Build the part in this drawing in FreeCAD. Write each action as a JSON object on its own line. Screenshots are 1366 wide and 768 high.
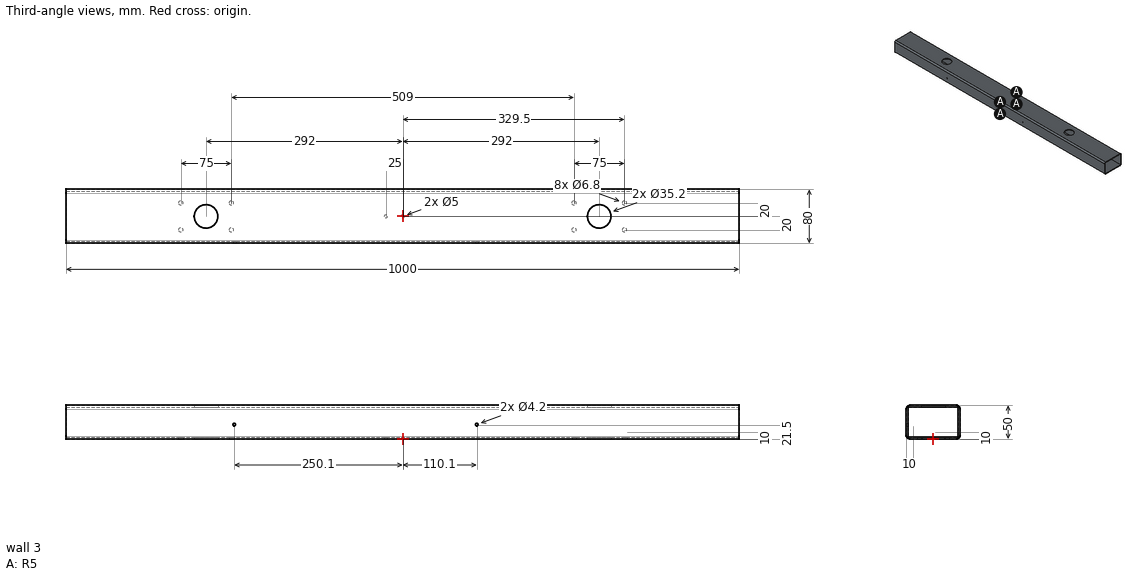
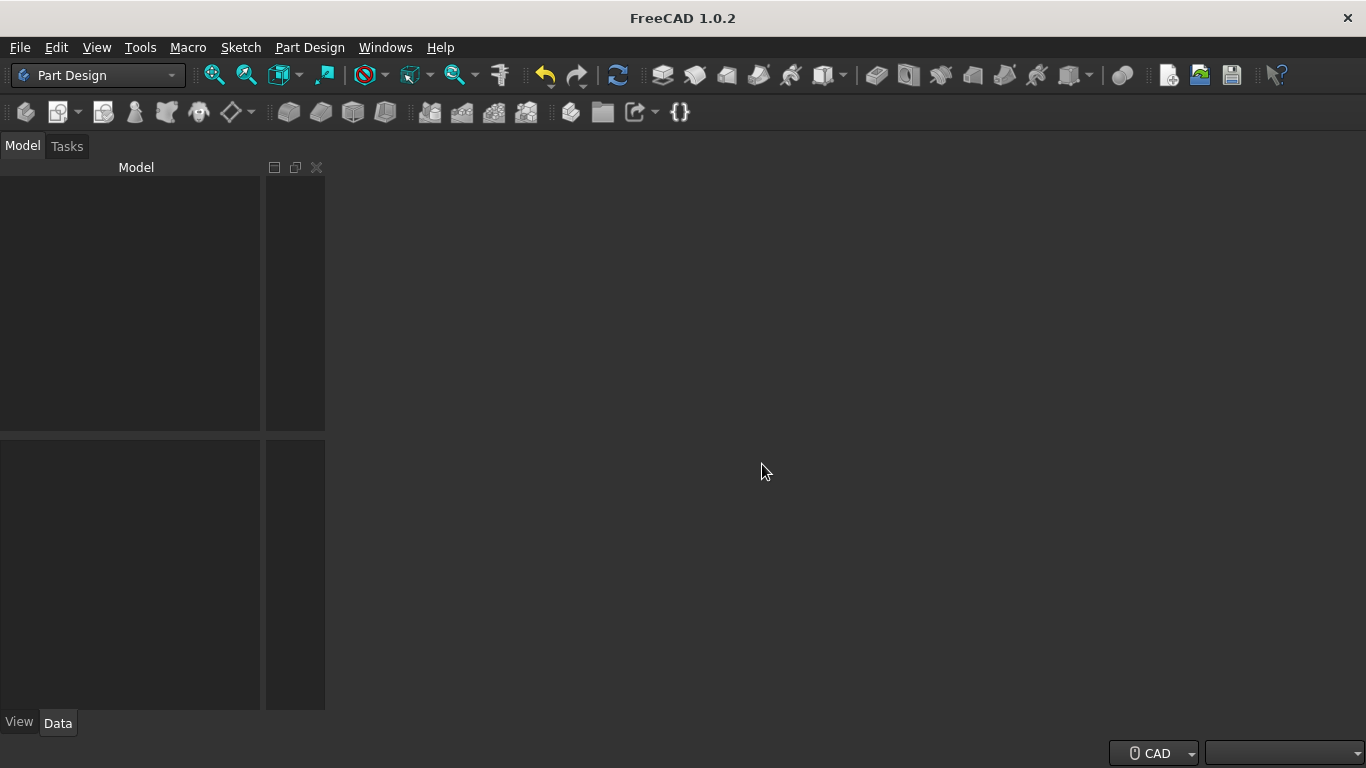
{"action": "key", "text": "ctrl+n"}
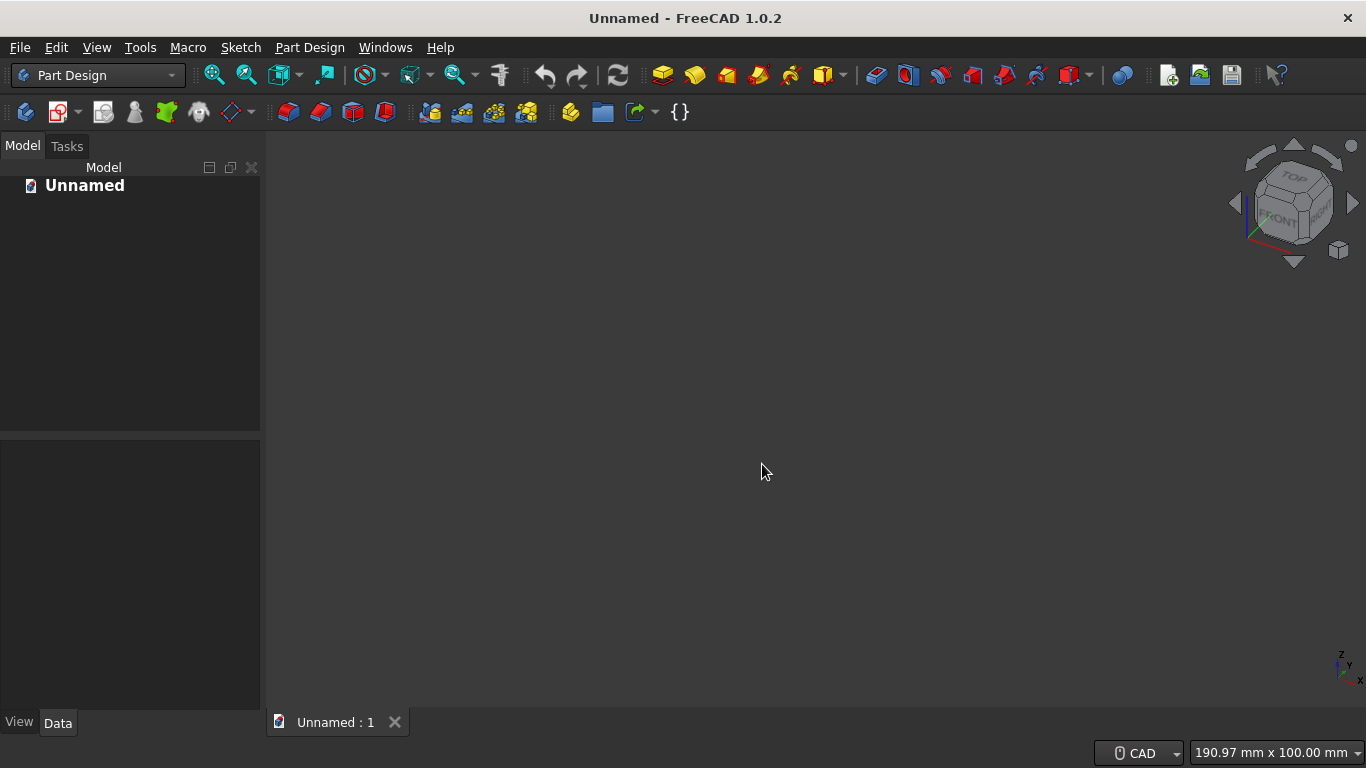
{"action": "left_click", "coordinate": [58, 112]}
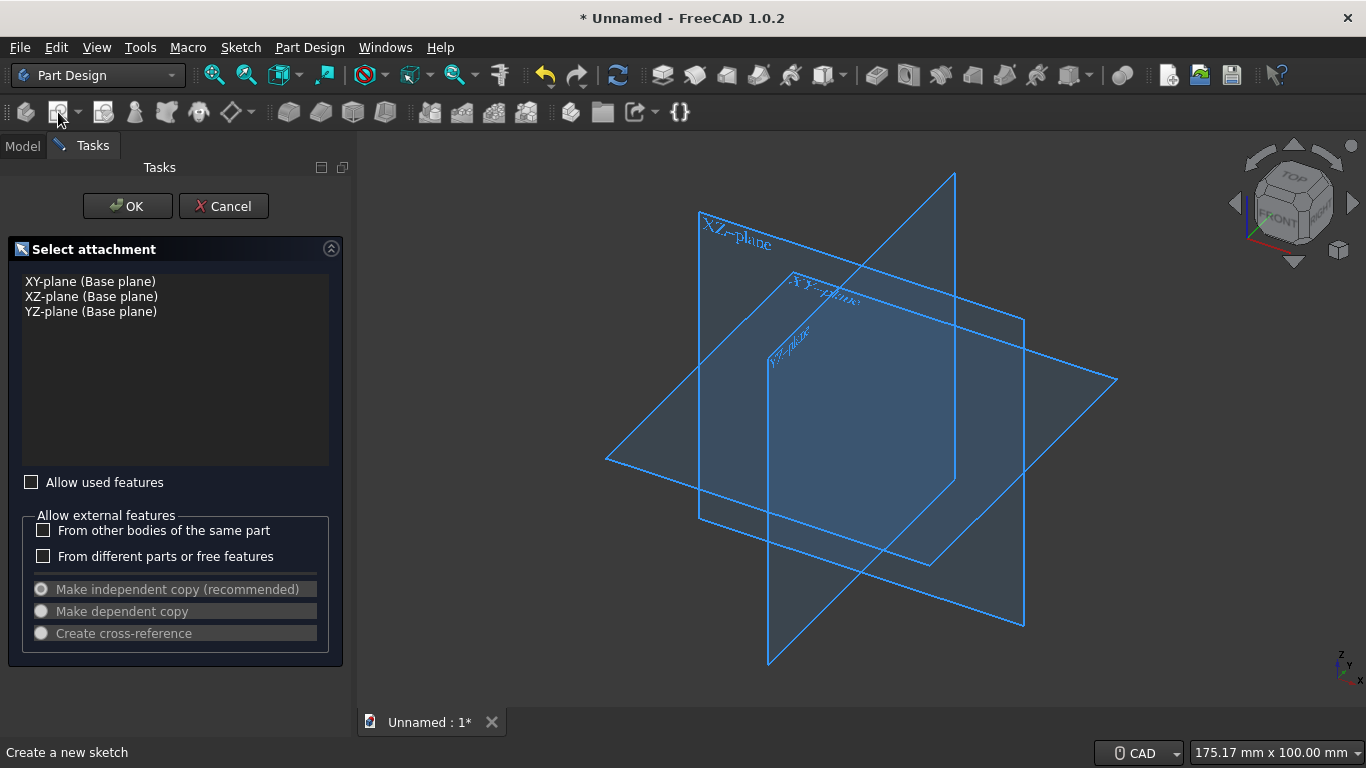
{"action": "left_click", "coordinate": [82, 282]}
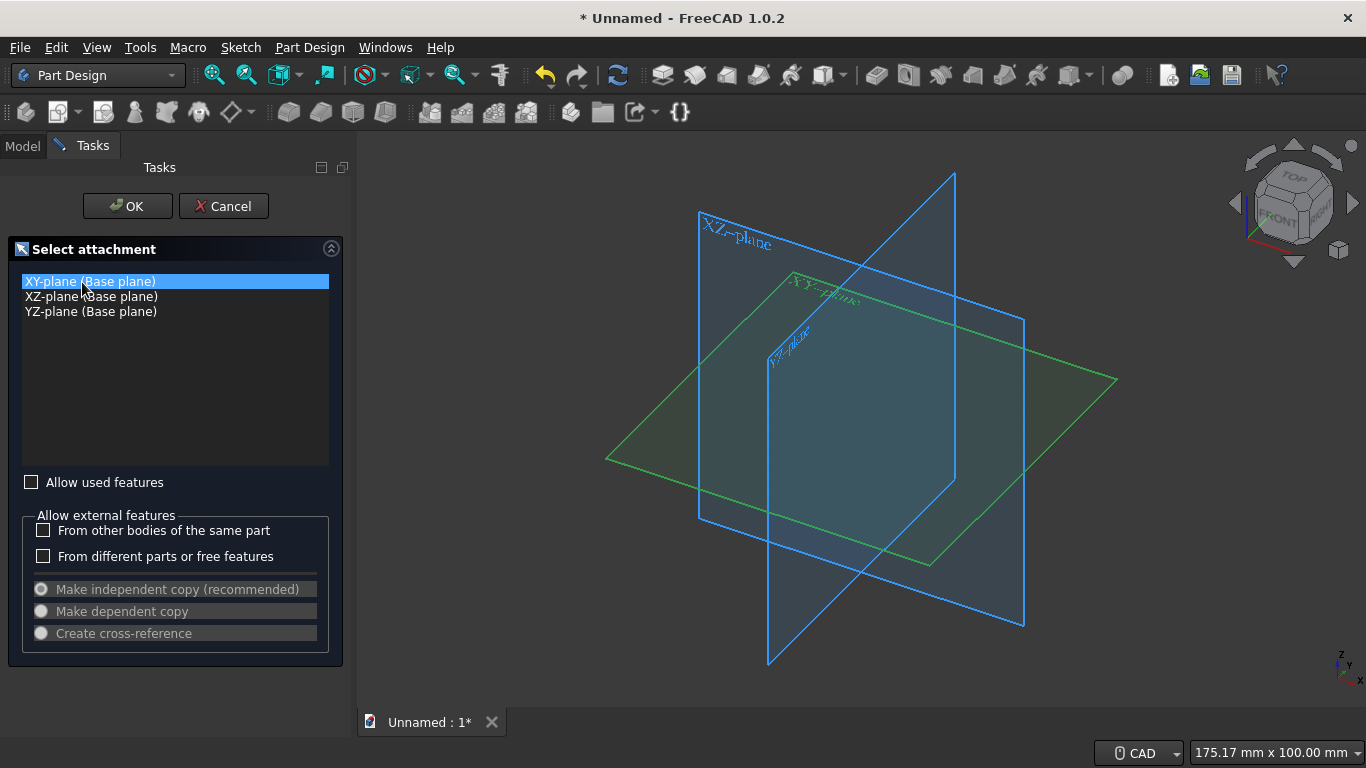
{"action": "left_click", "coordinate": [128, 206]}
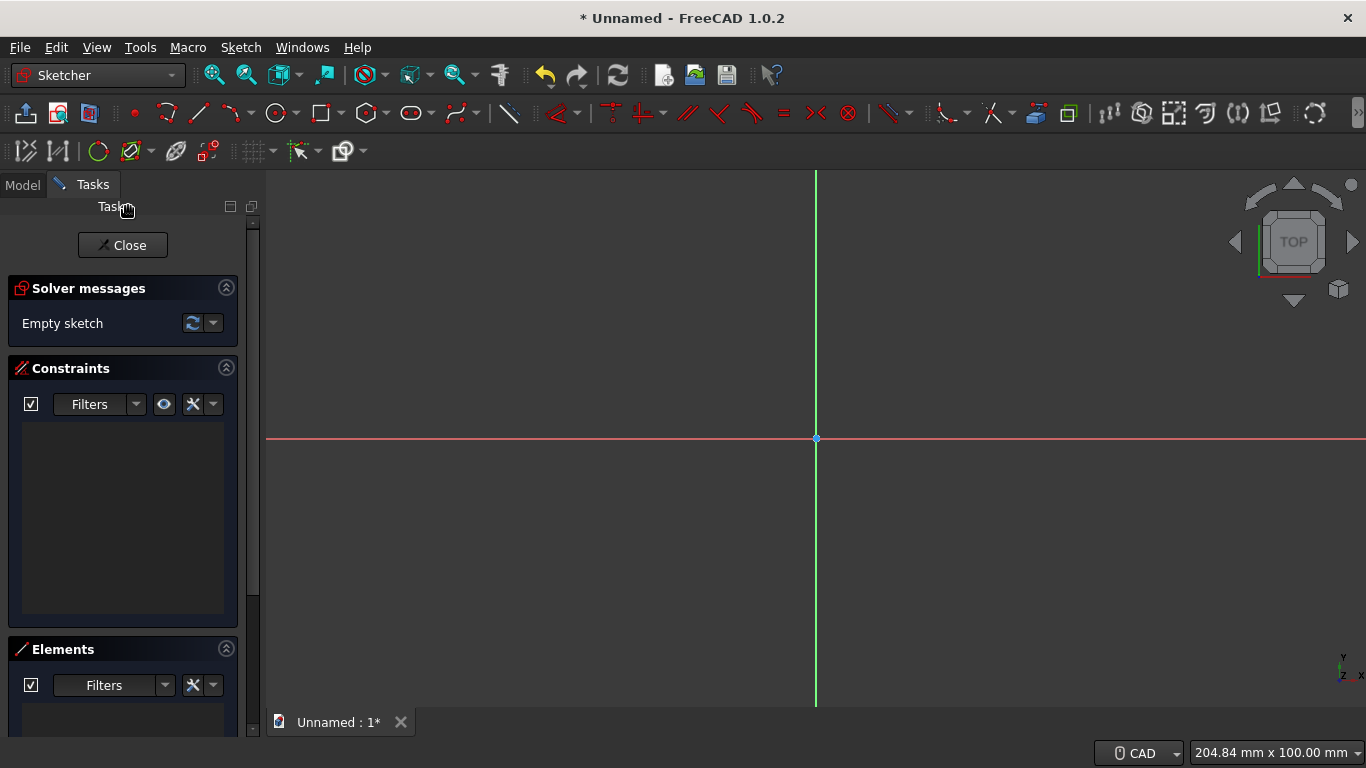
{"action": "scroll", "coordinate": [739, 439], "scroll_direction": "down", "scroll_amount": 11}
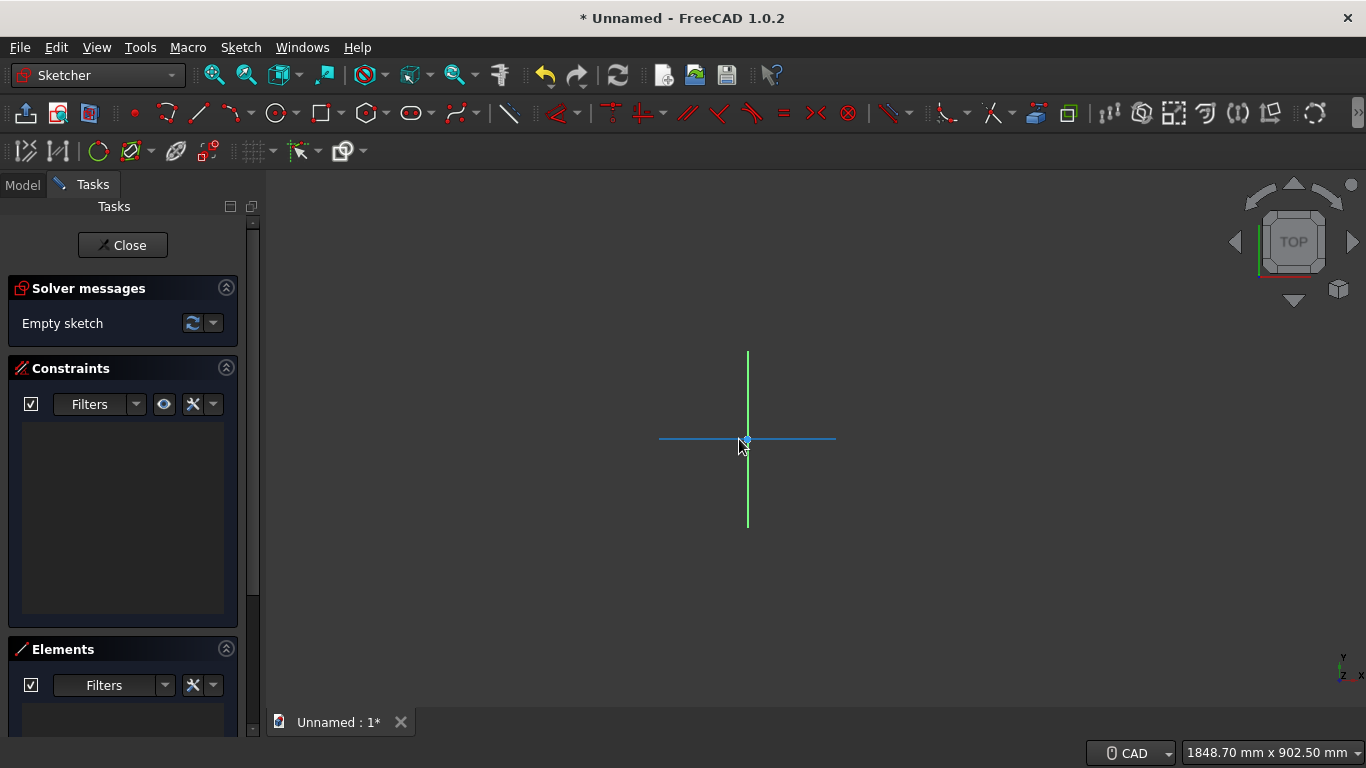
{"action": "key", "text": "g v"}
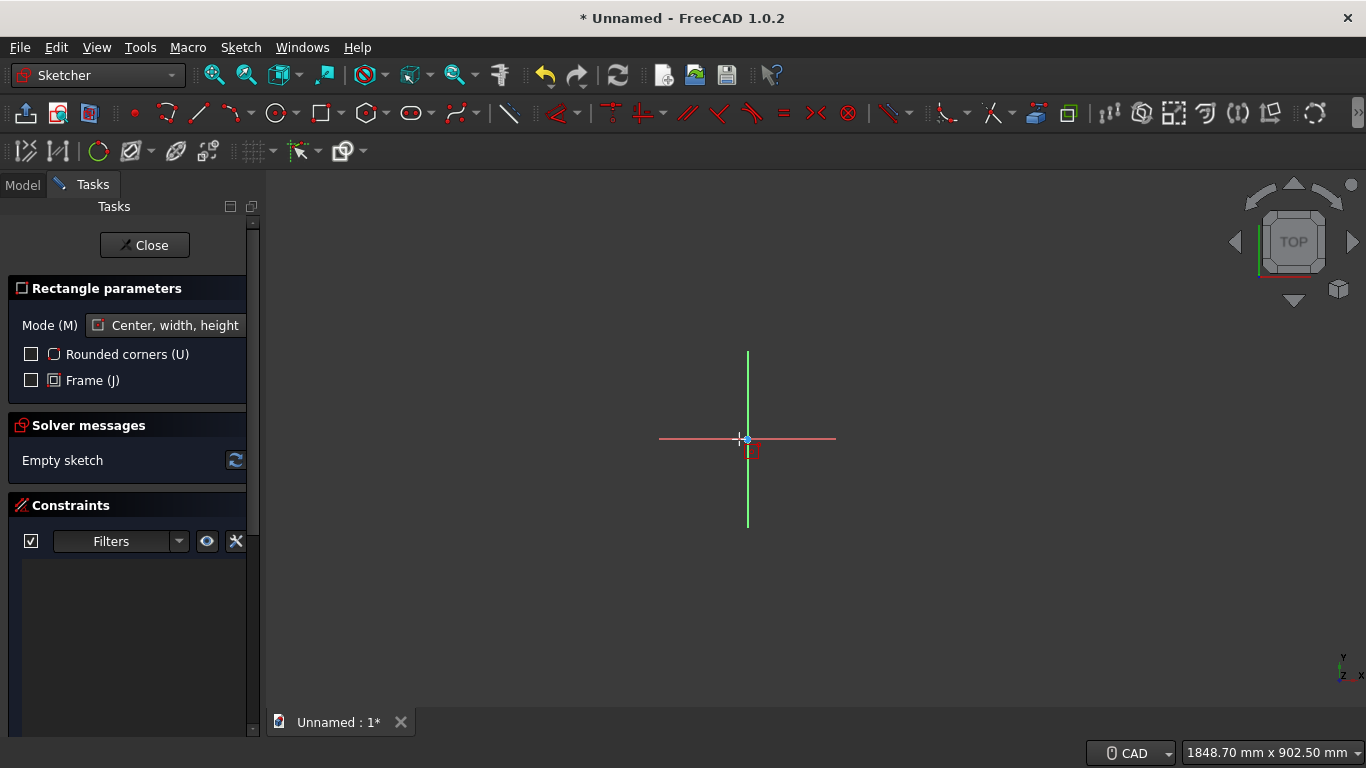
{"action": "left_click", "coordinate": [748, 439]}
{"action": "mouse_move", "coordinate": [1045, 416]}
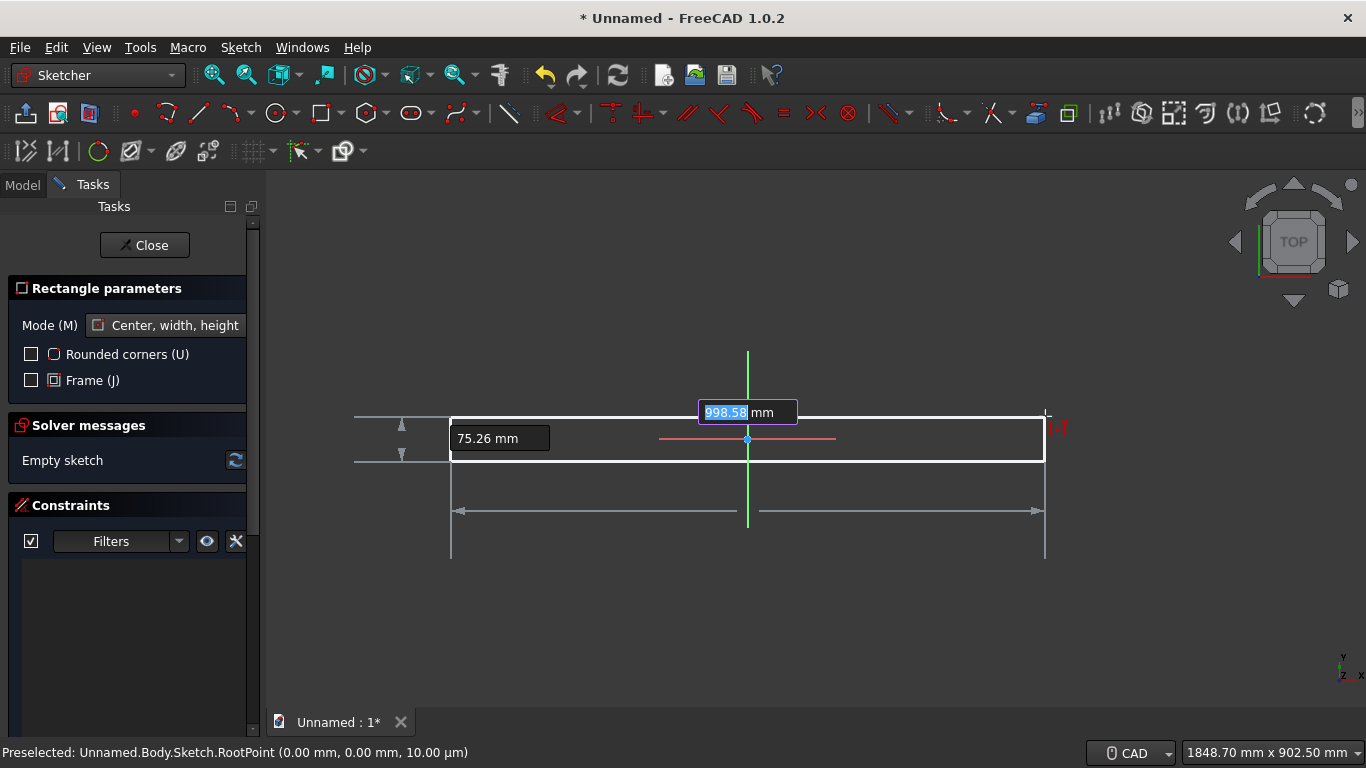
{"action": "type", "text": "1000"}
{"action": "key", "text": "Tab"}
{"action": "type", "text": "80"}
{"action": "key", "text": "Return"}
{"action": "key", "text": "Escape"}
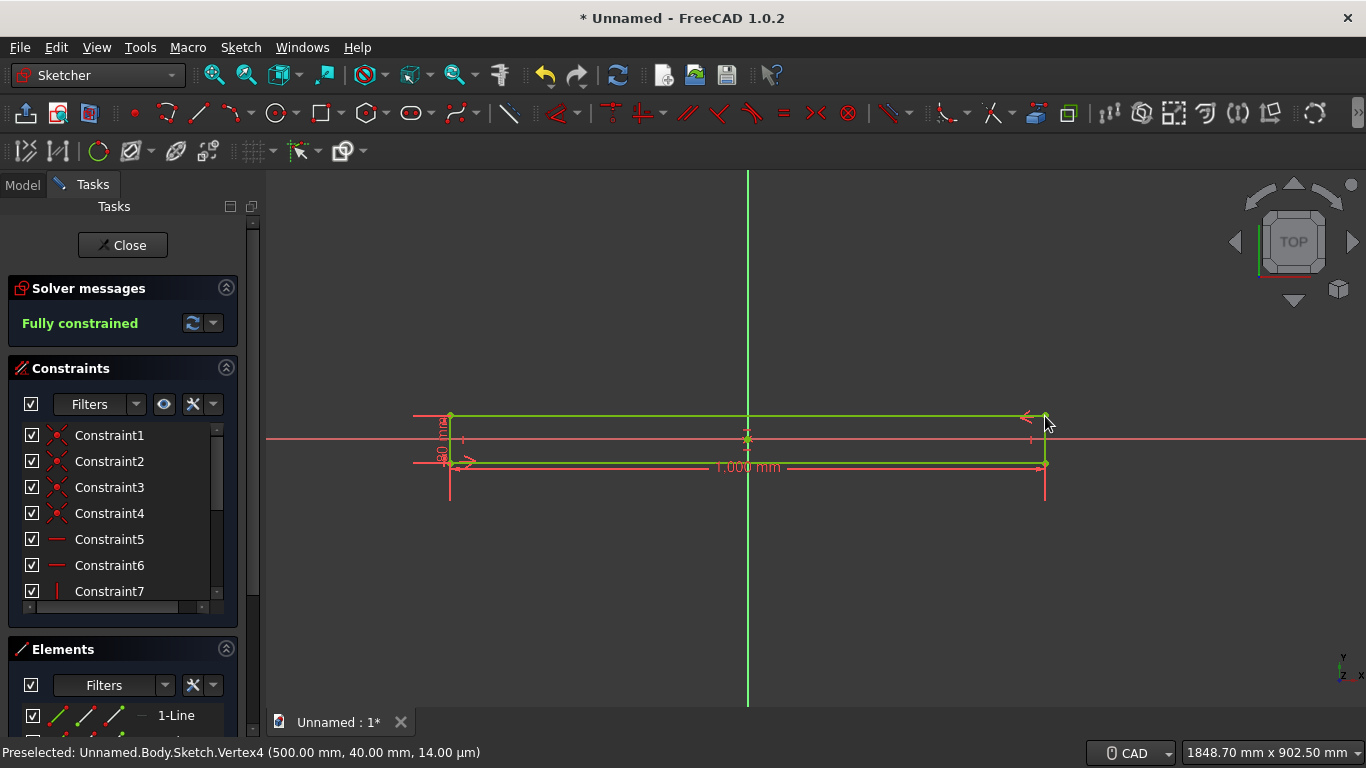
{"action": "left_click", "coordinate": [123, 245]}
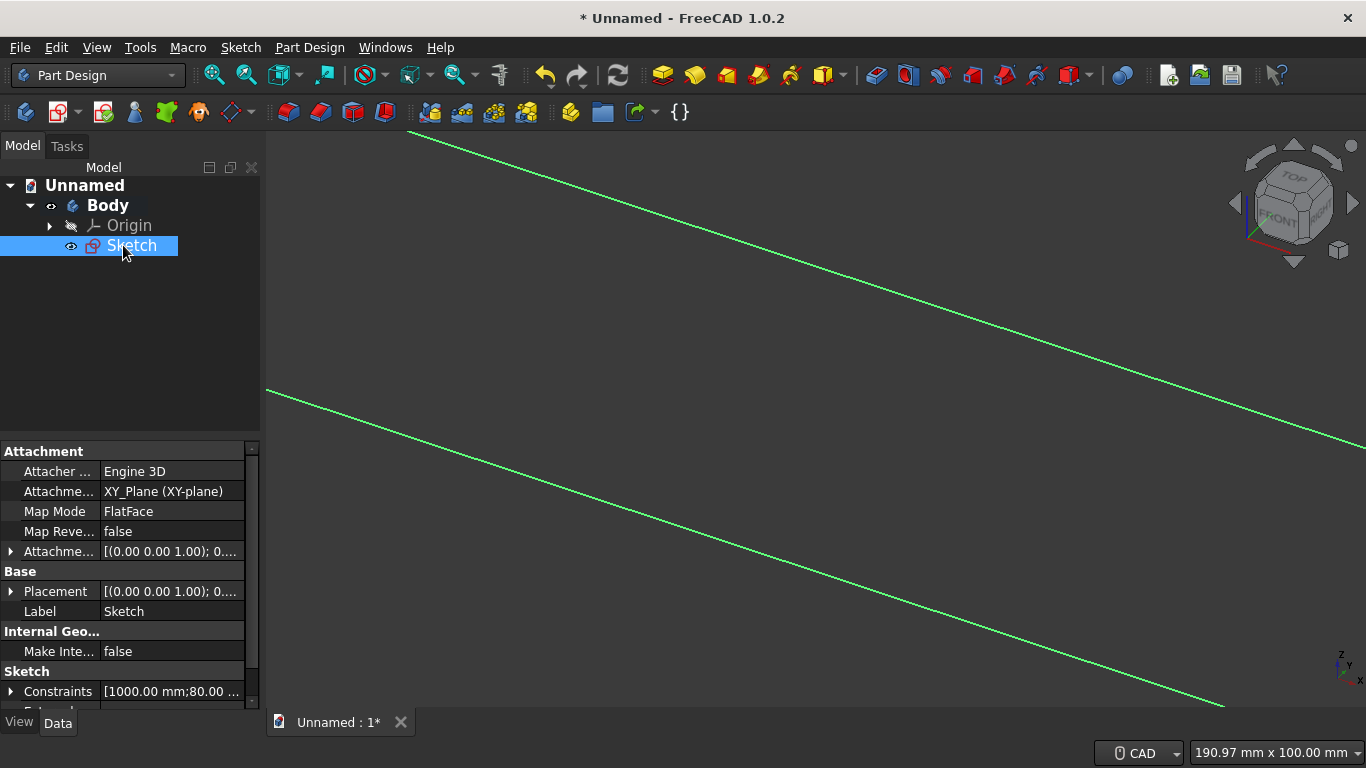
{"action": "left_click", "coordinate": [664, 76]}